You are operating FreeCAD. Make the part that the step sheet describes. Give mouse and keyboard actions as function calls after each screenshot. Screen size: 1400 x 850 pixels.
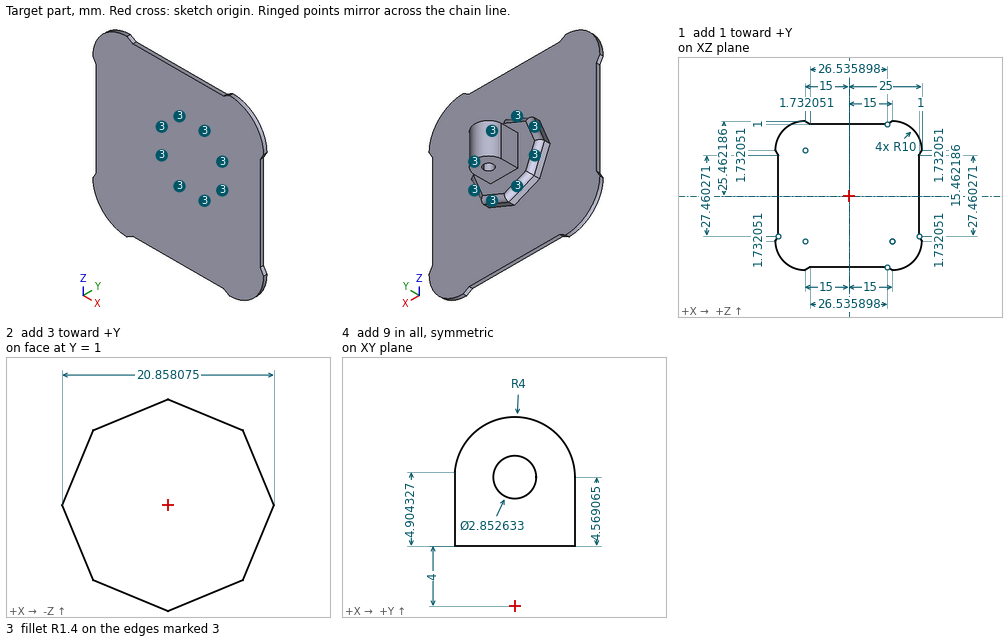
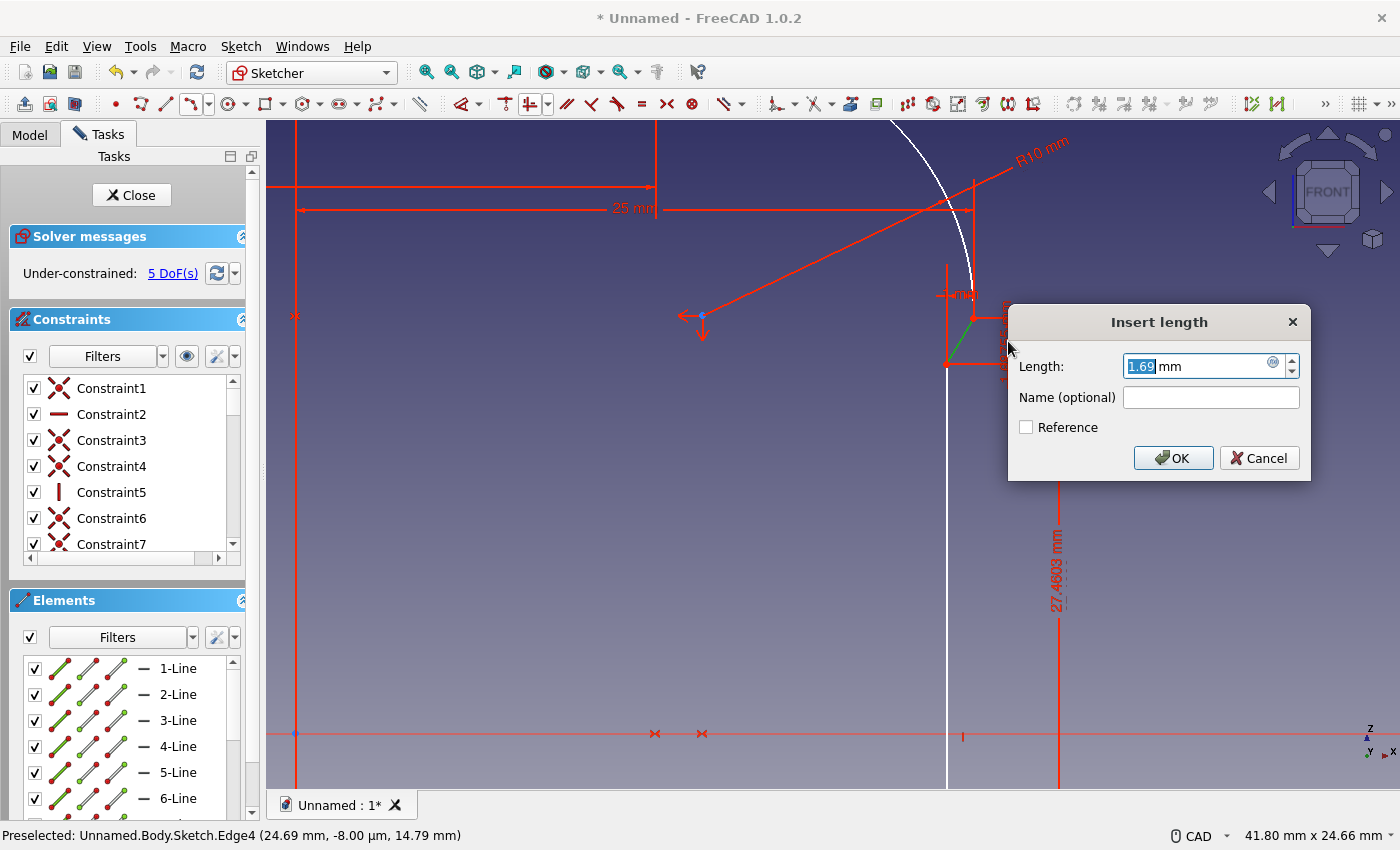
text(1.732051)
key(Return)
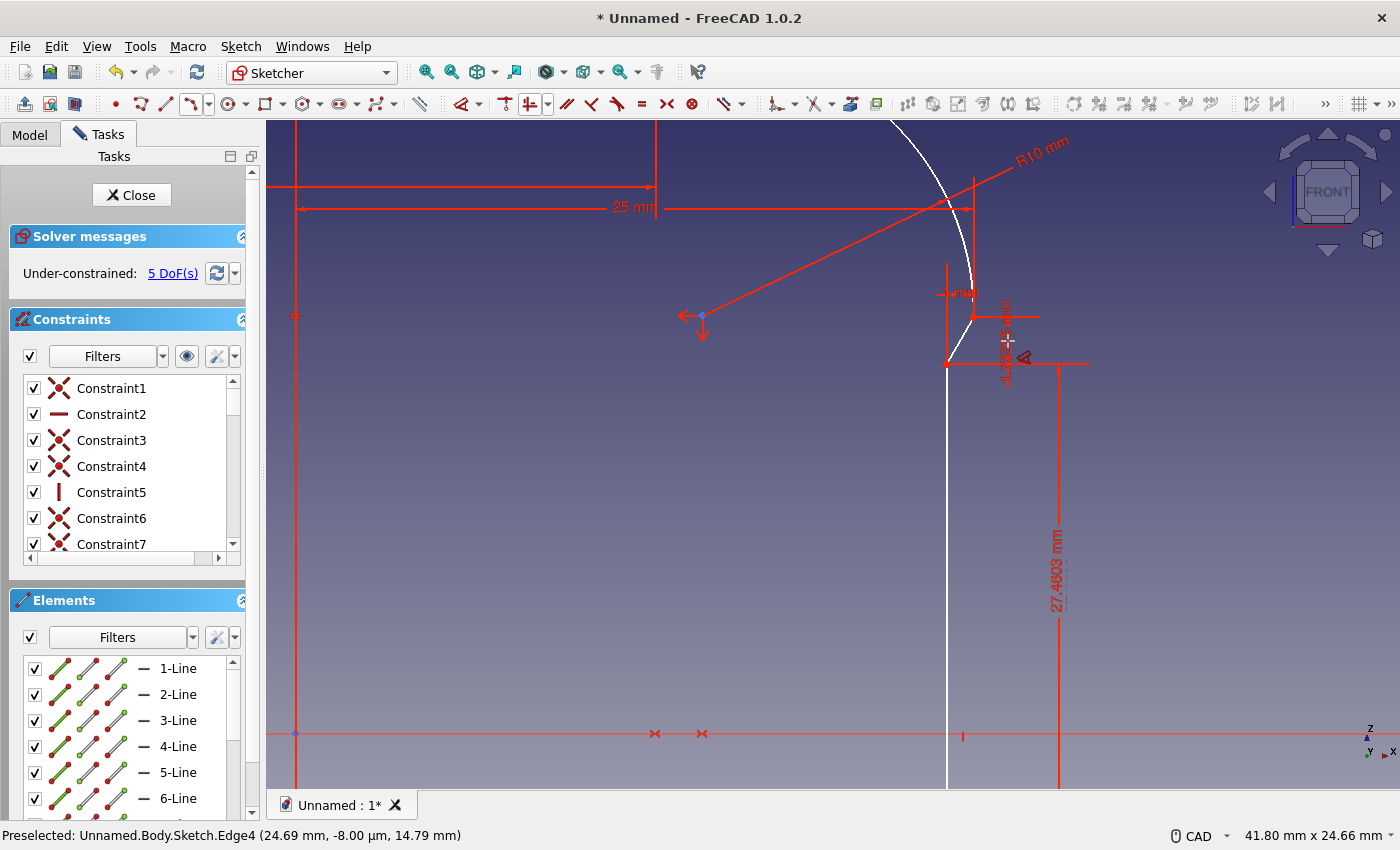
scroll(967, 334, down, 6)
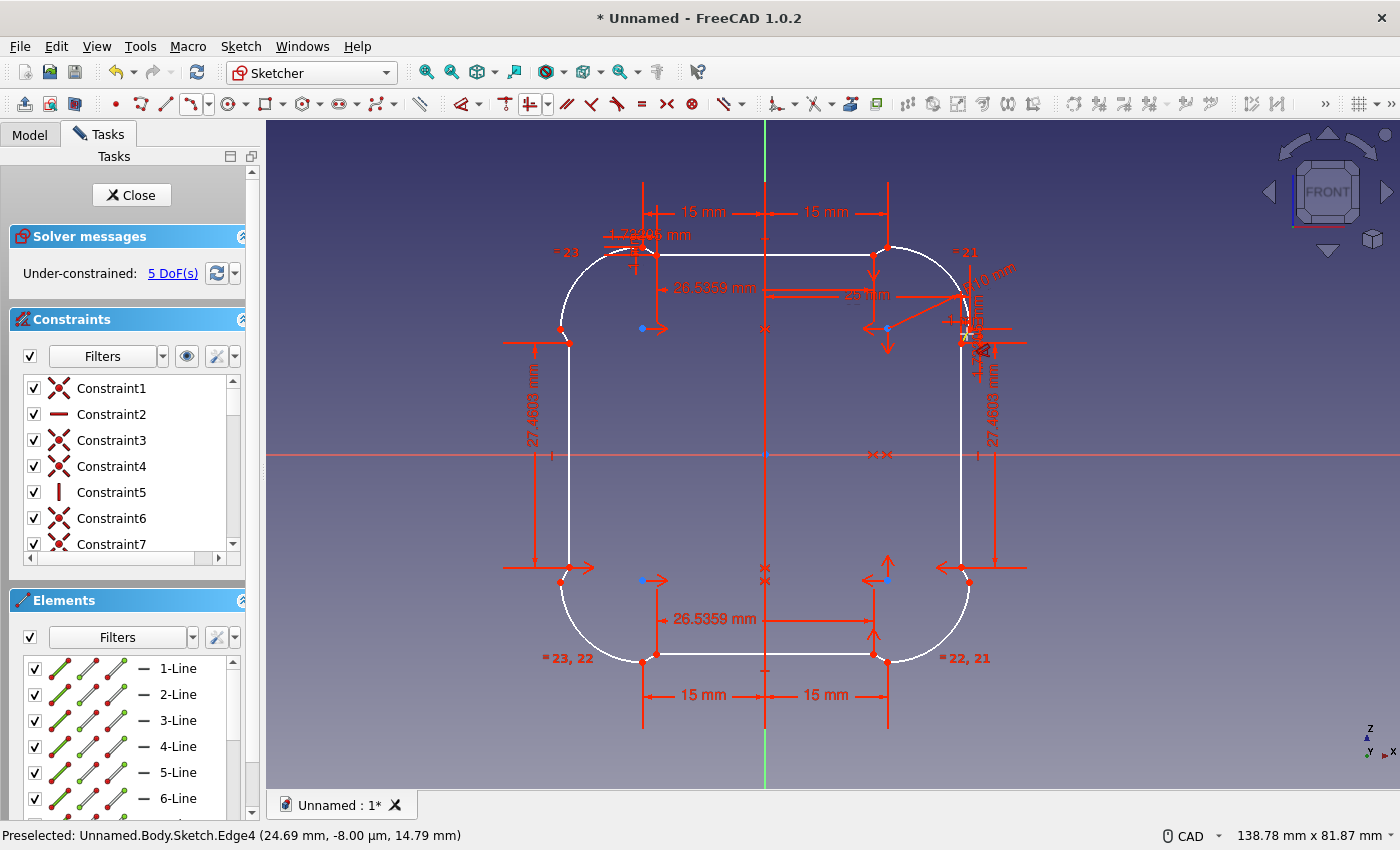
scroll(964, 572, up, 6)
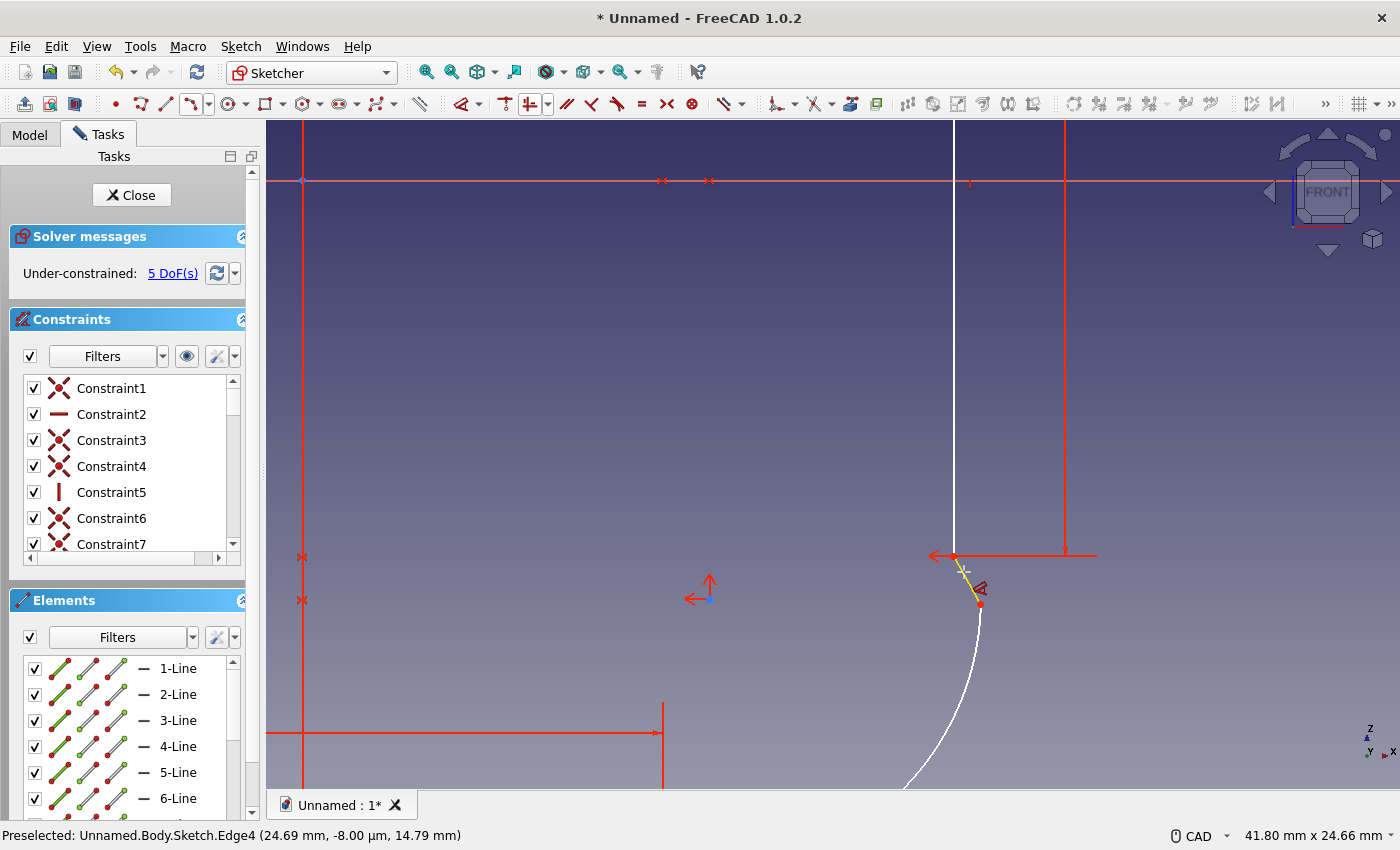
click(962, 571)
click(1015, 580)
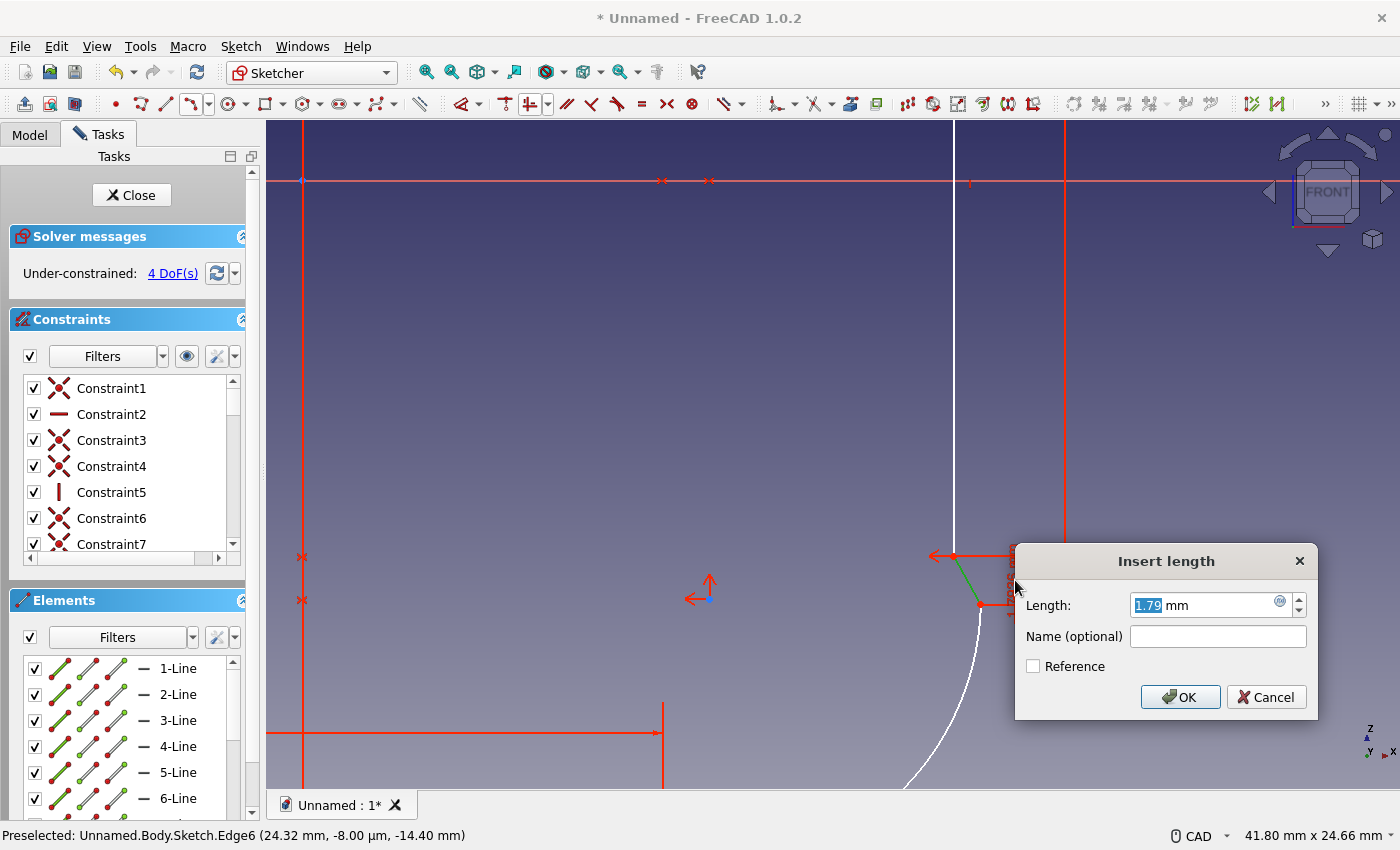
text(1.732051)
key(Return)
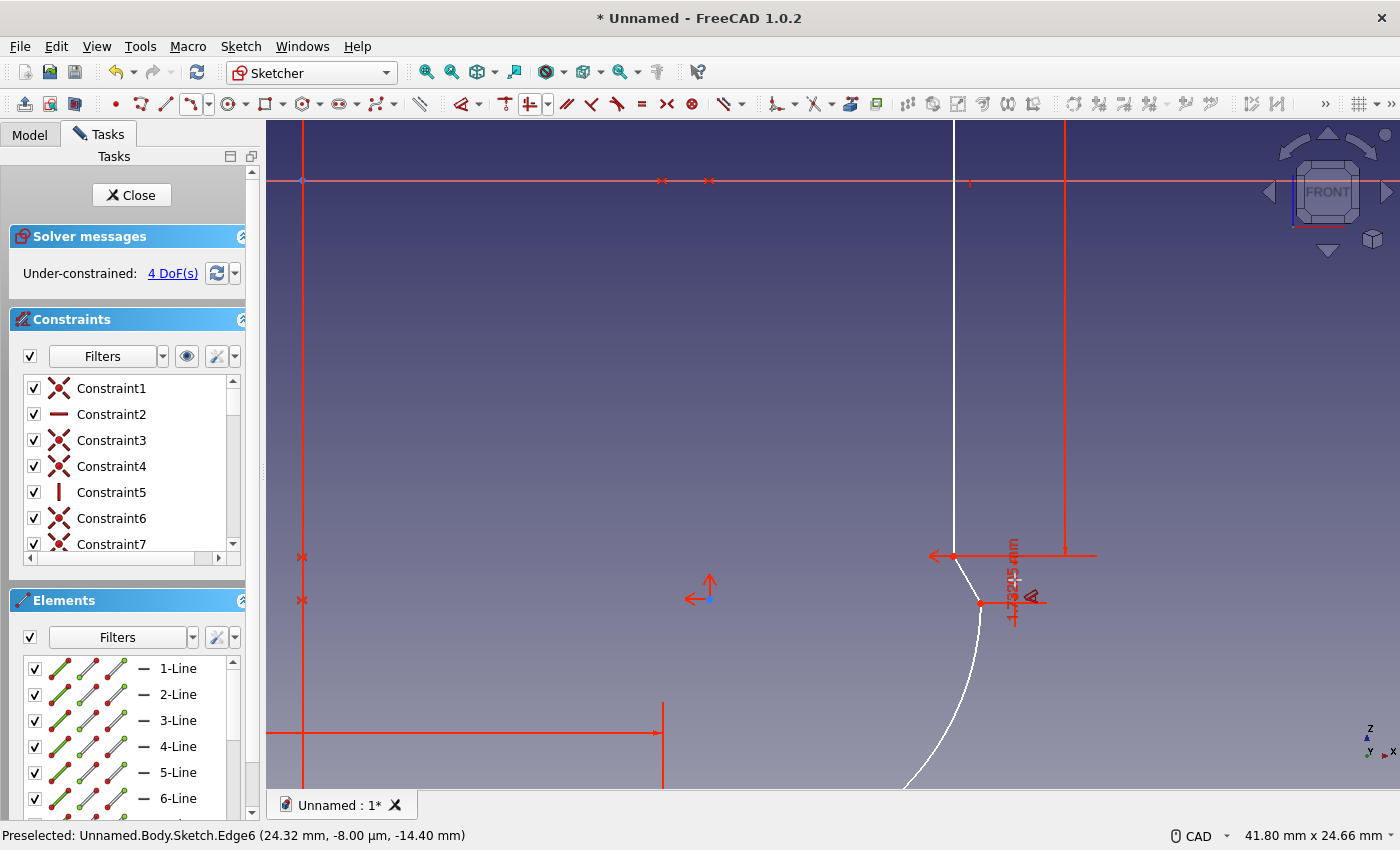
scroll(964, 572, down, 6)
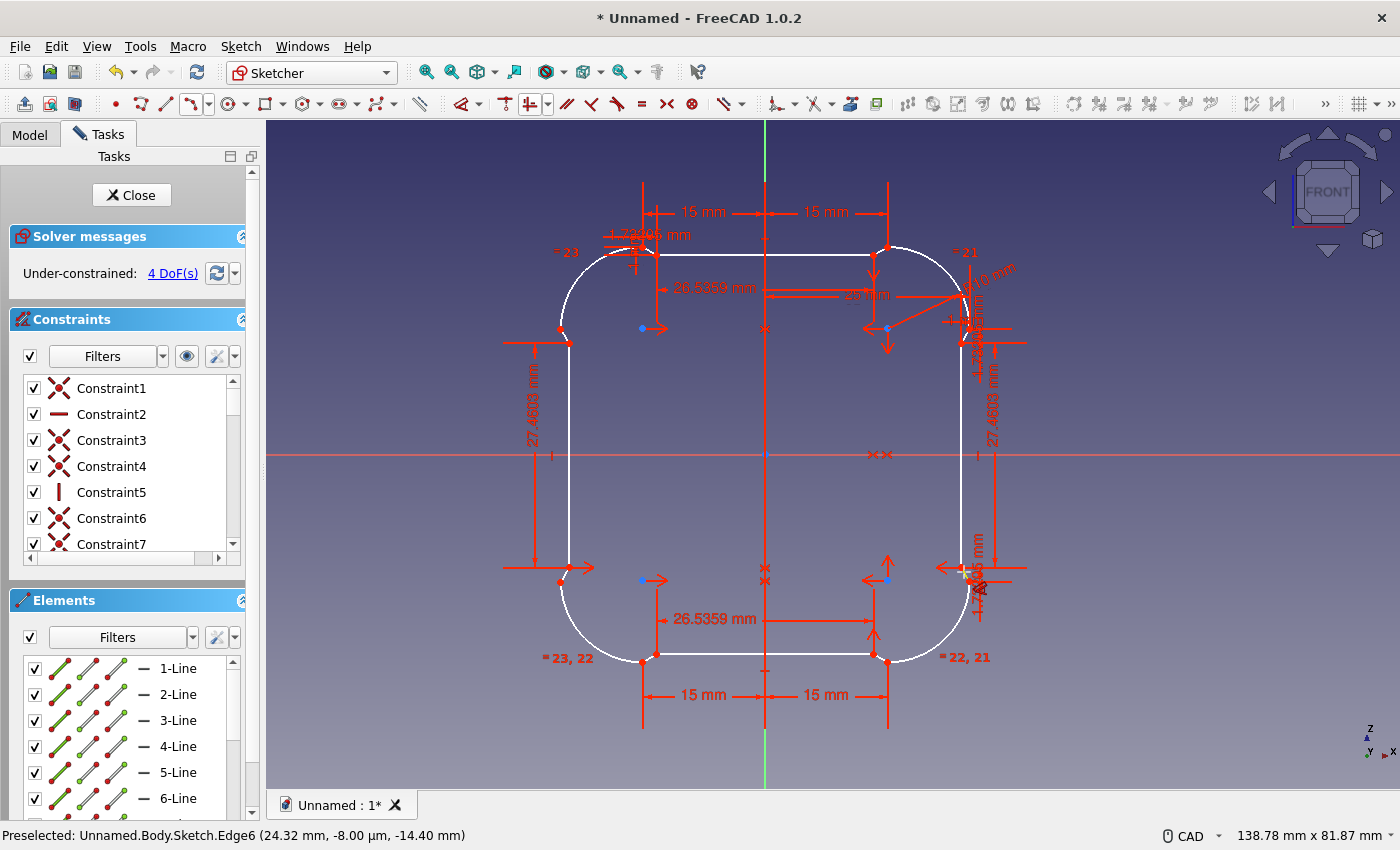
scroll(563, 578, up, 6)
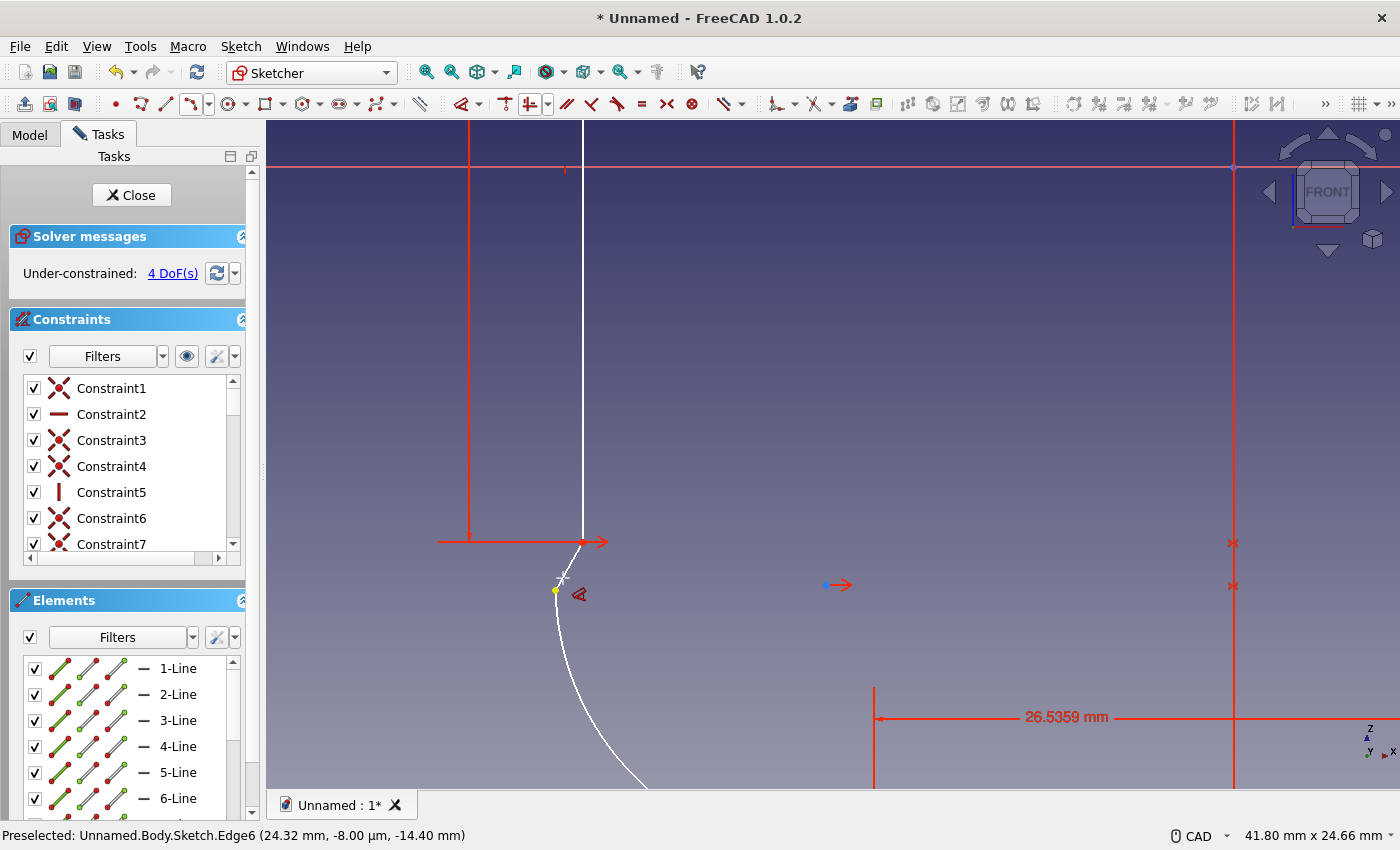
click(564, 576)
click(522, 566)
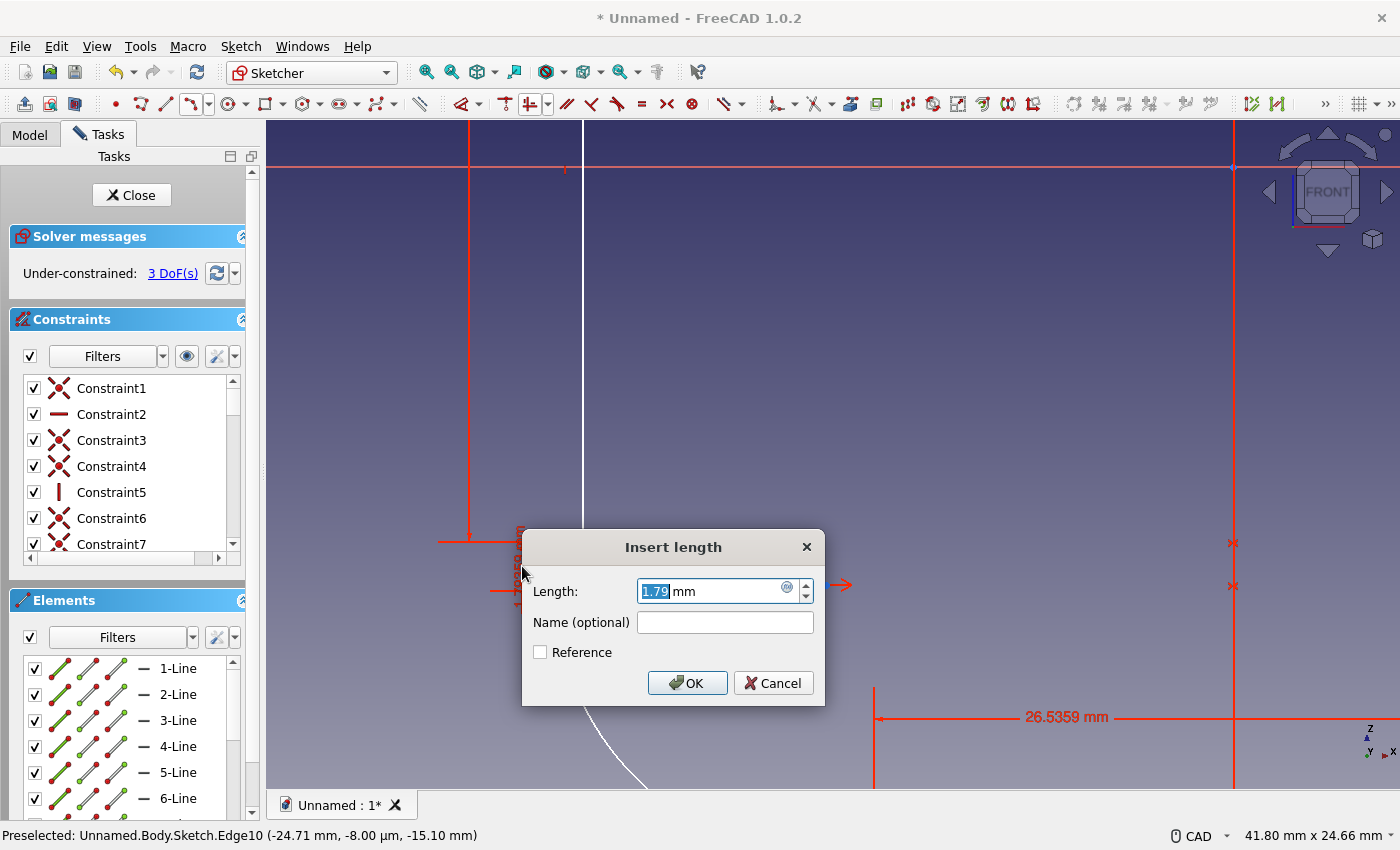
text(1.732051)
key(Return)